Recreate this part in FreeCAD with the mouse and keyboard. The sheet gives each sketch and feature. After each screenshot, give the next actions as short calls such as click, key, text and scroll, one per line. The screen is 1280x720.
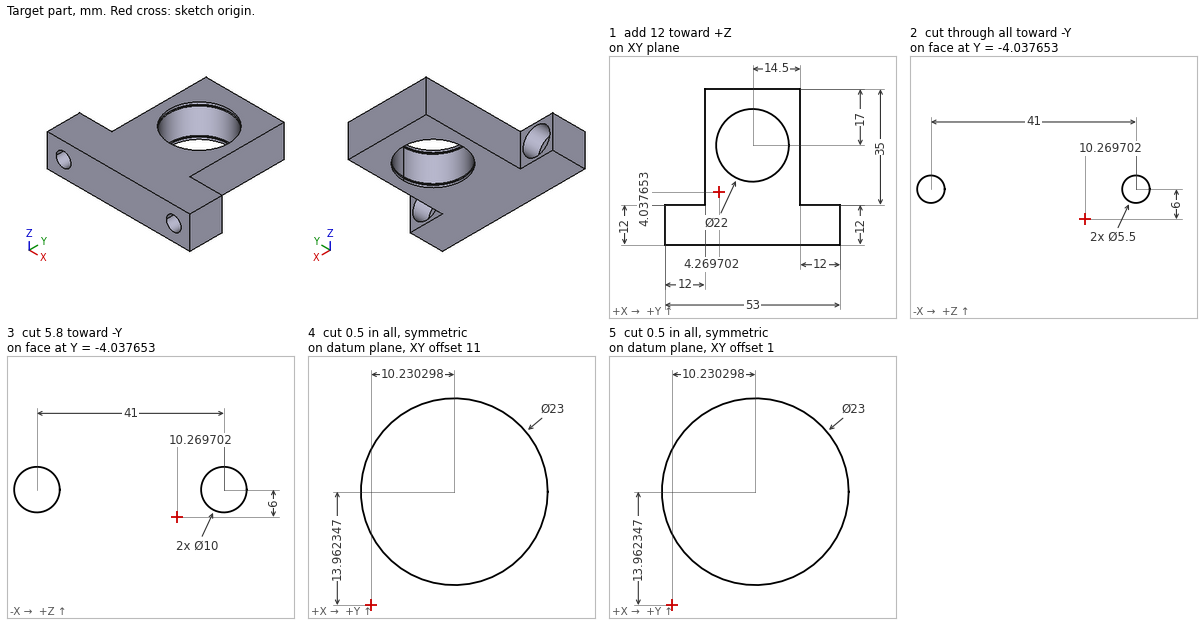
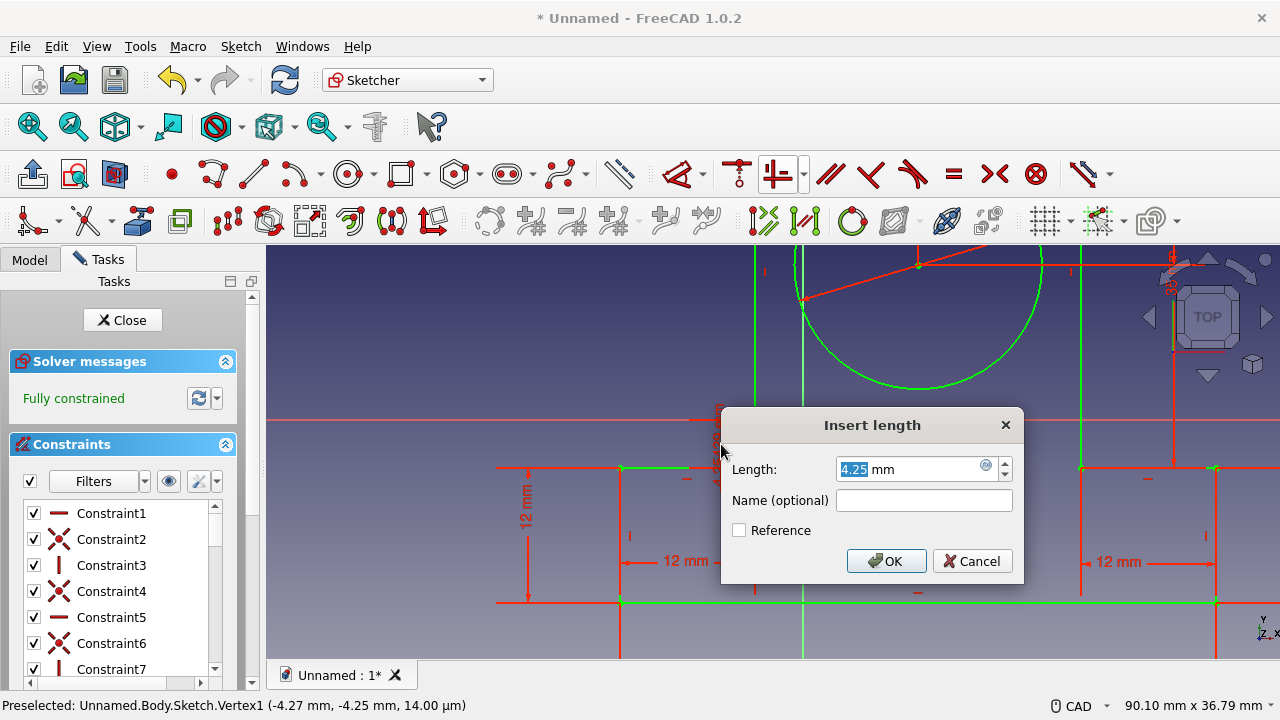
text(4.037653)
key(Return)
key(Escape)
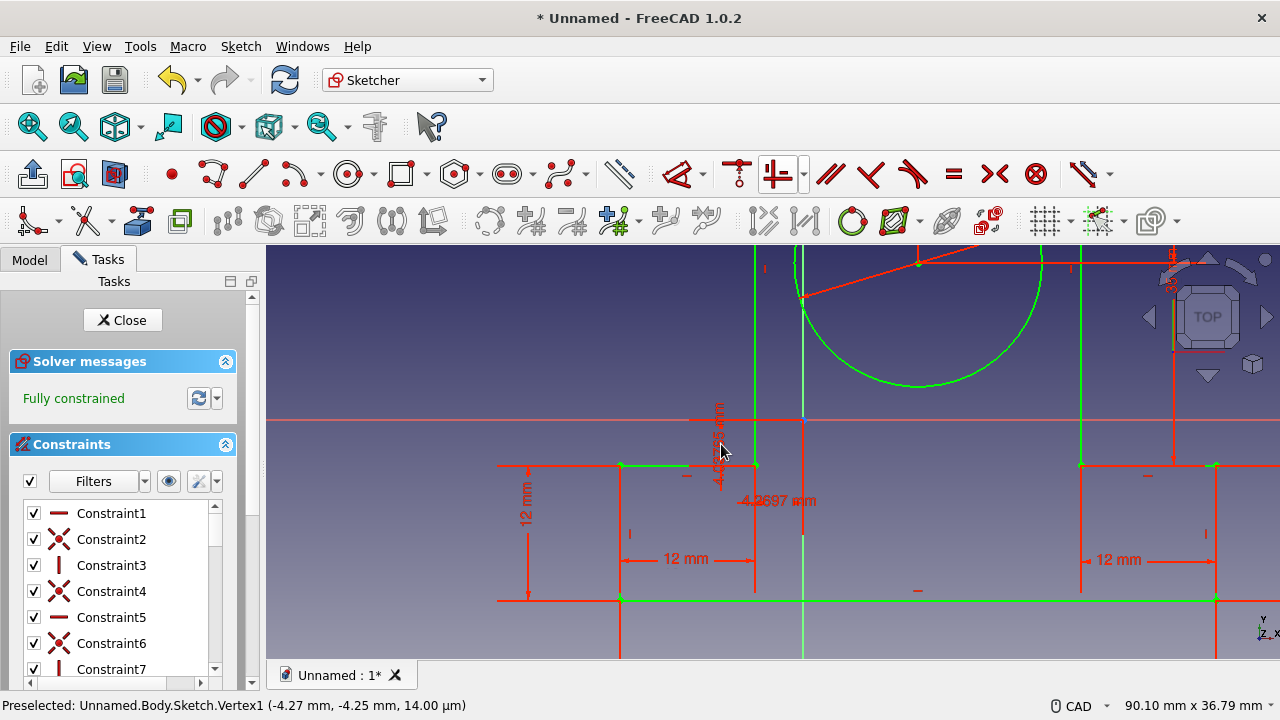
click(123, 320)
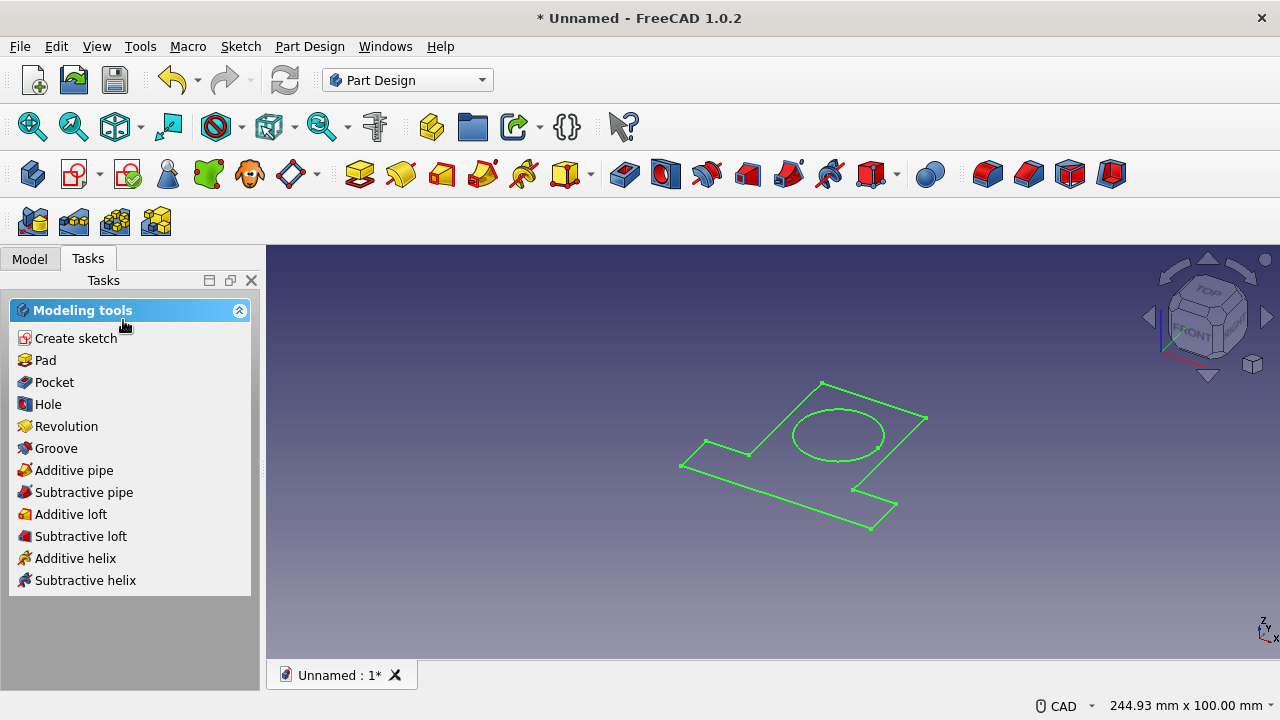
click(360, 174)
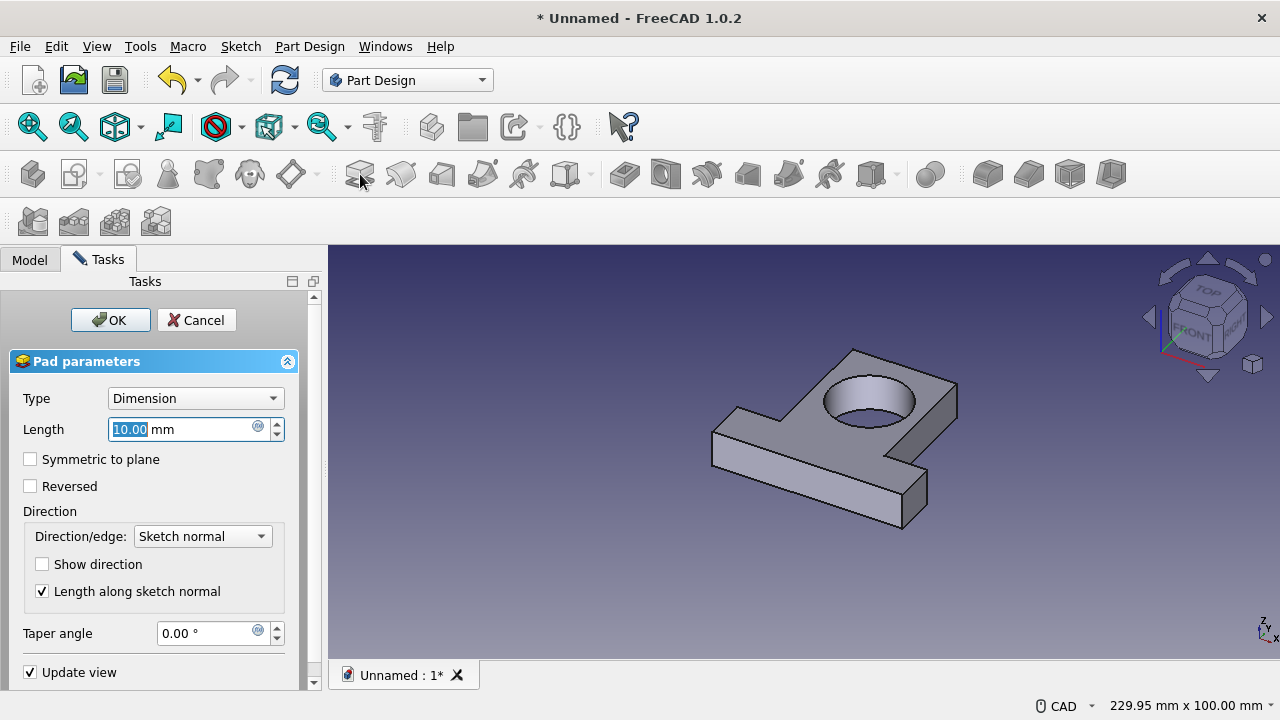
text(12)
key(Tab)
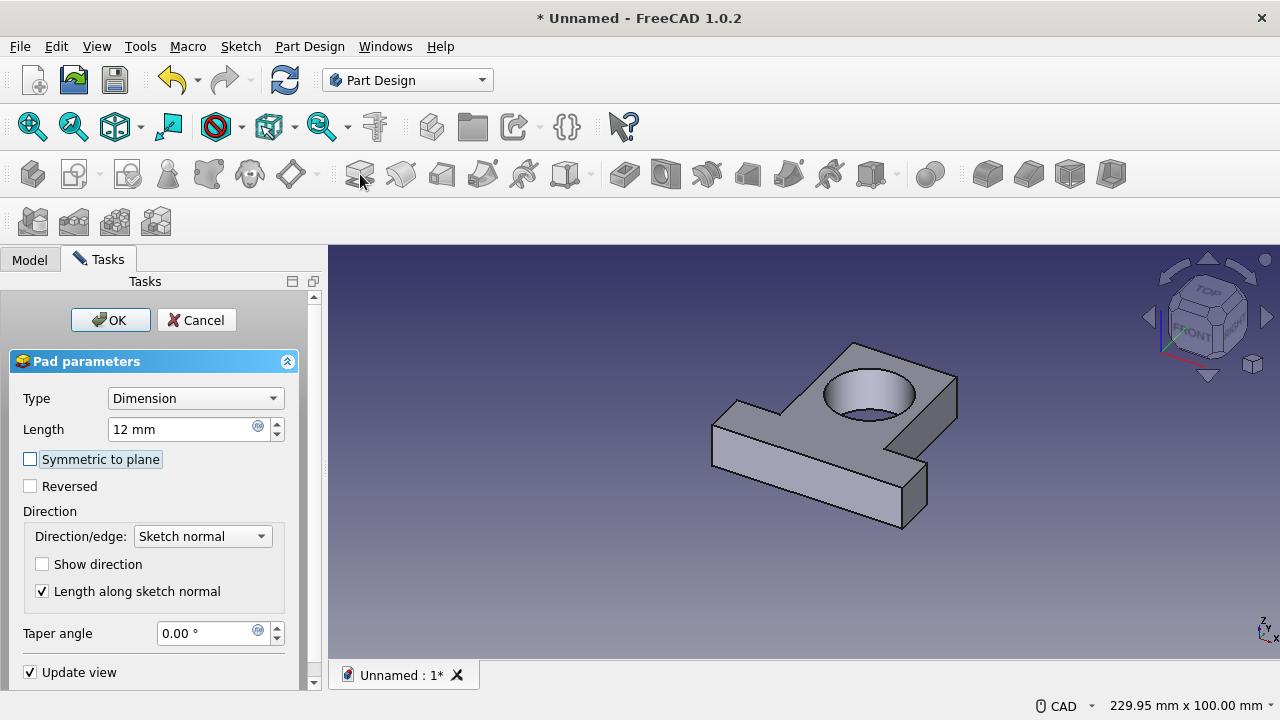
click(111, 320)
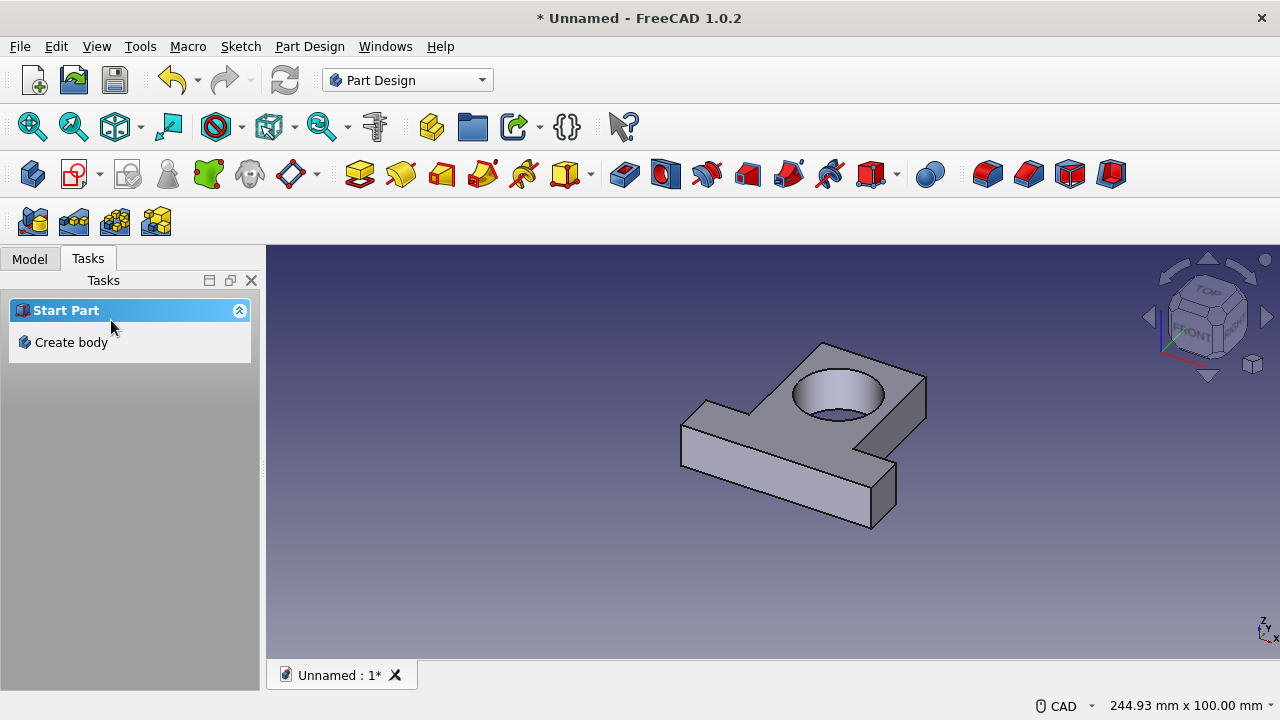
key(4)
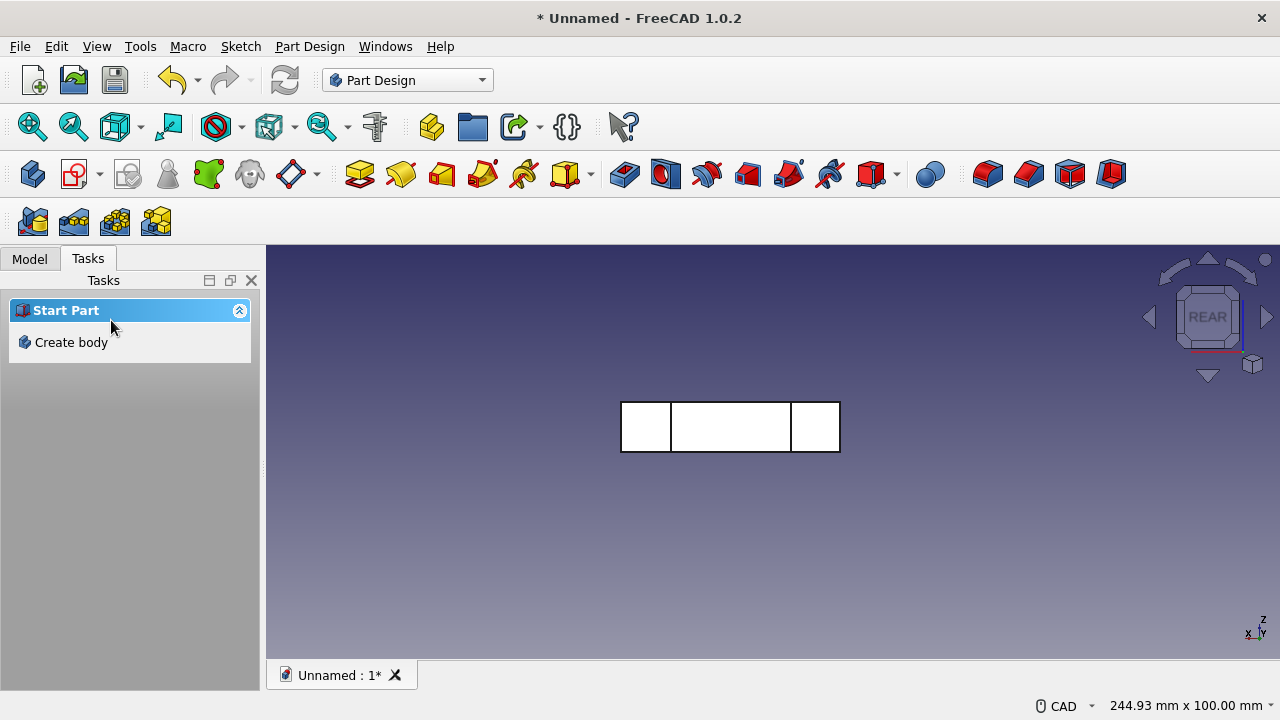
click(33, 128)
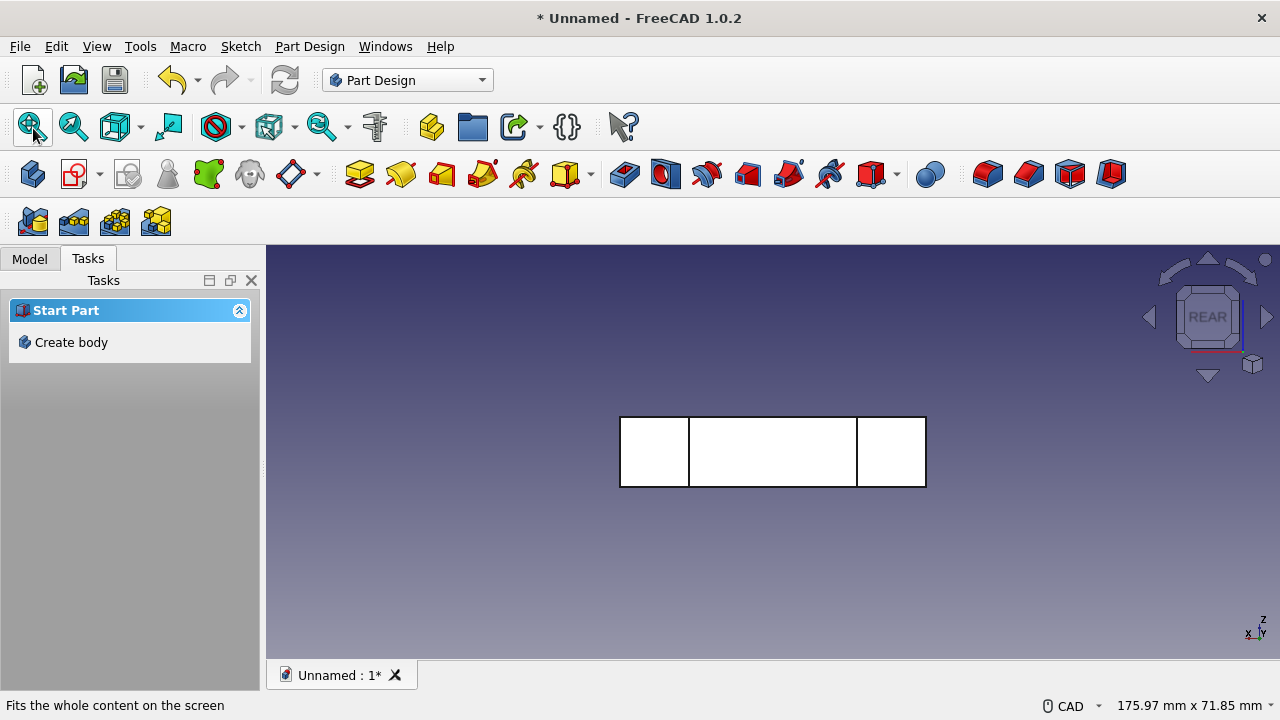
click(655, 451)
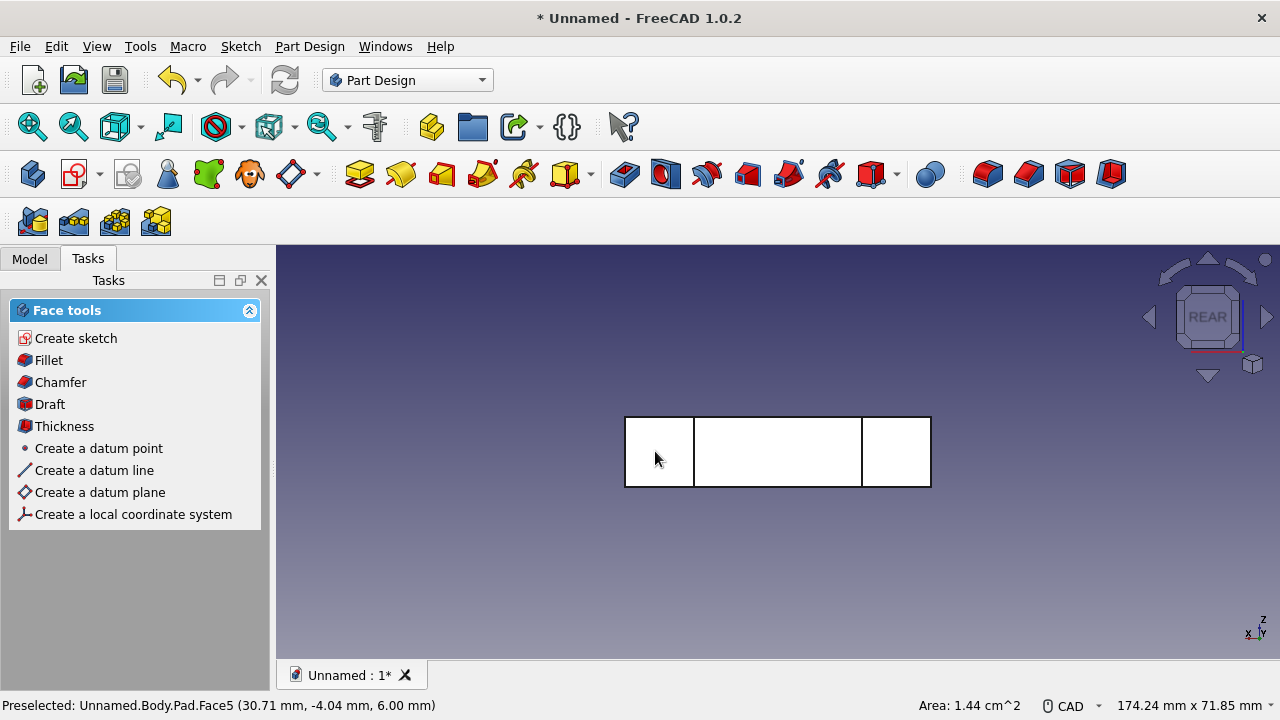
click(74, 174)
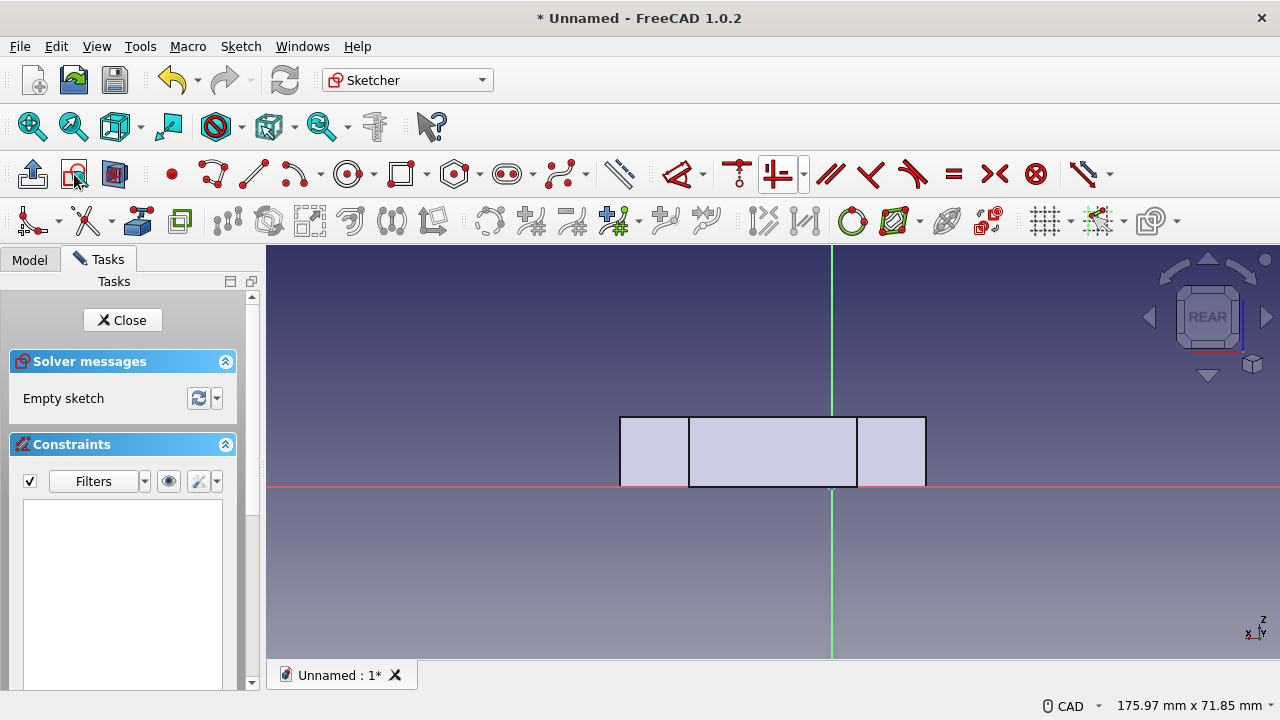
scroll(829, 469, up, 4)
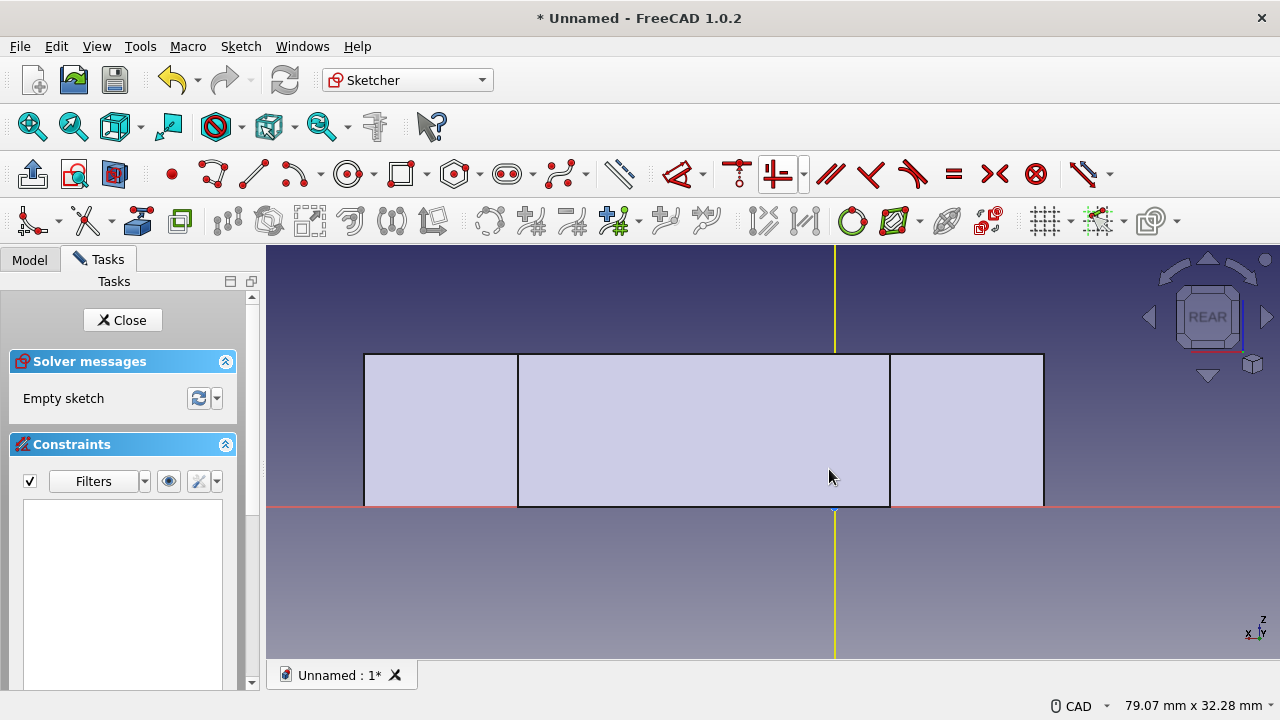
click(348, 174)